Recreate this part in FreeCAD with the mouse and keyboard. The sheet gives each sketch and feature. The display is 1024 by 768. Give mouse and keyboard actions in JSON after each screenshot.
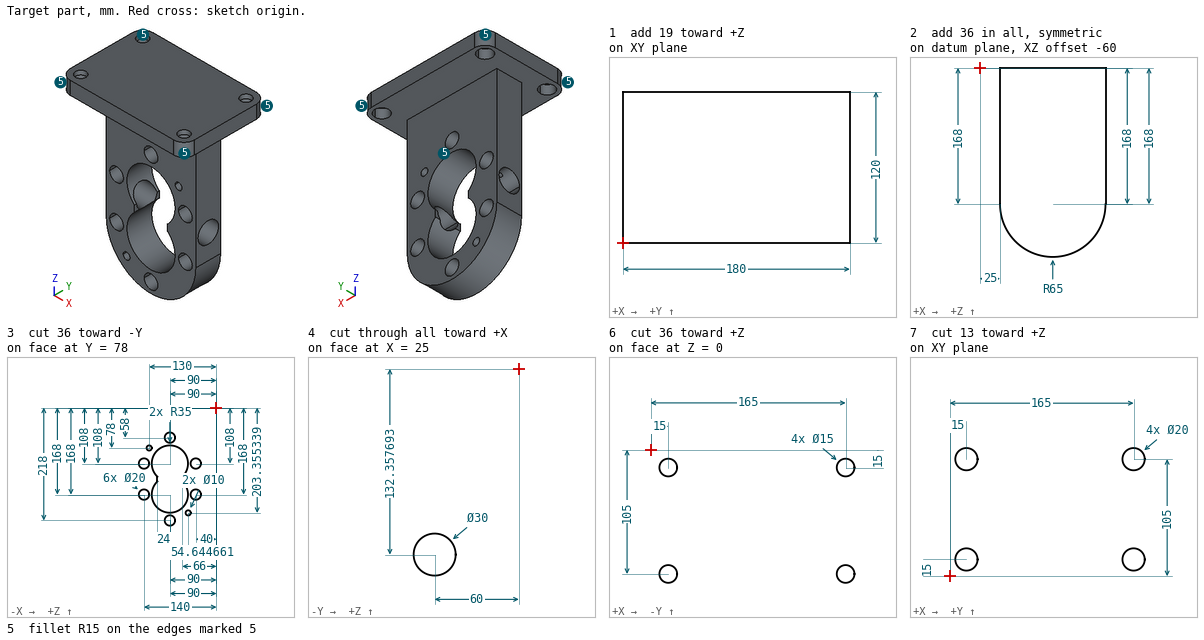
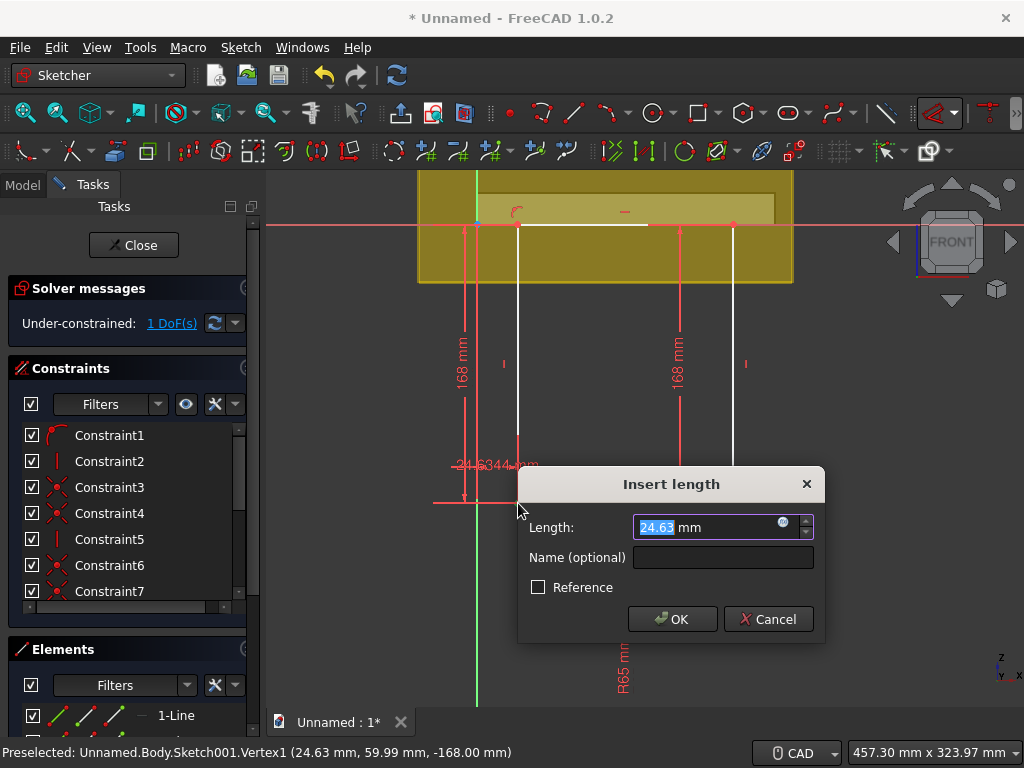
{"action": "type", "text": "25"}
{"action": "key", "text": "Return"}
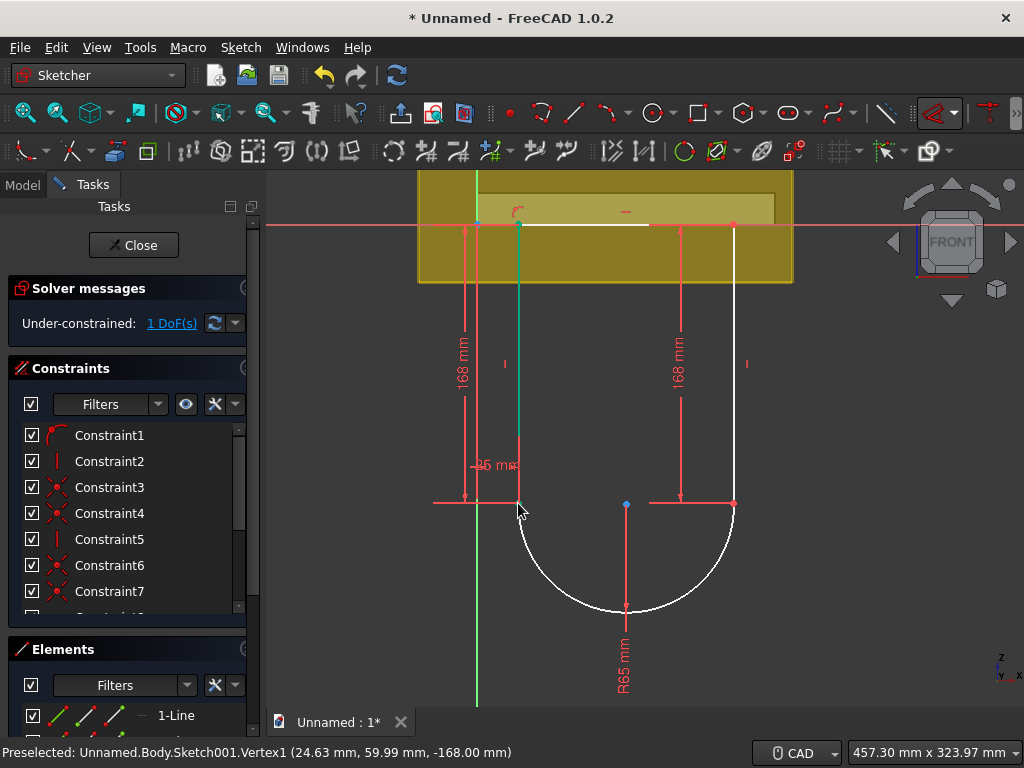
{"action": "left_click", "coordinate": [626, 505]}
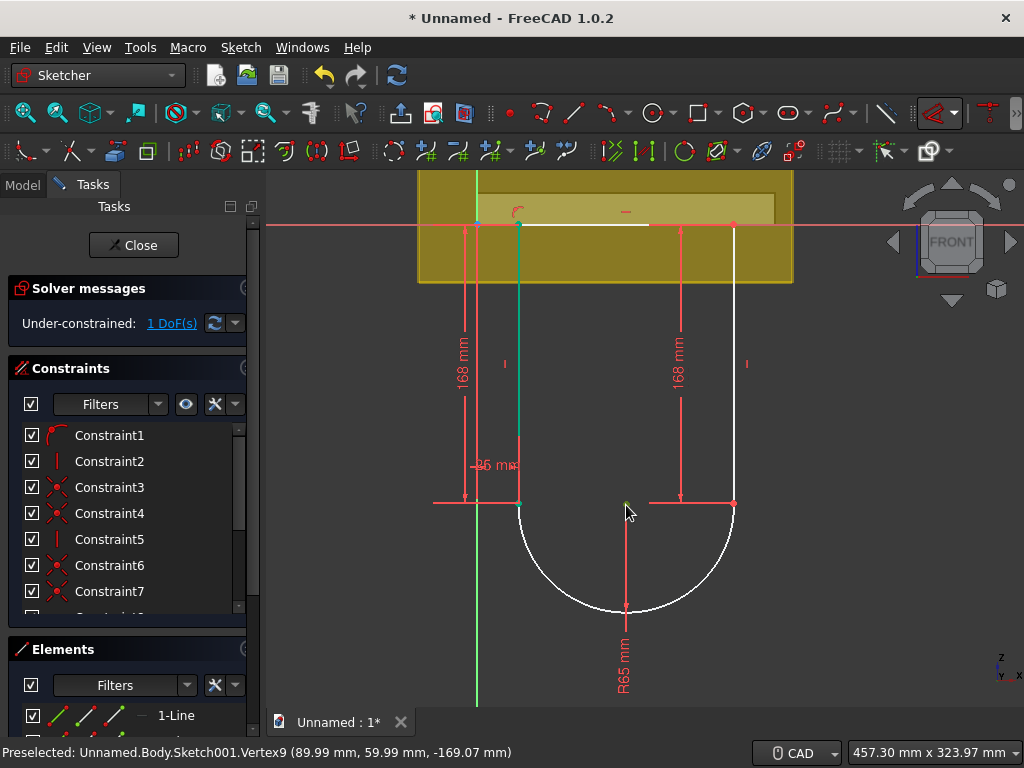
{"action": "left_click", "coordinate": [956, 114]}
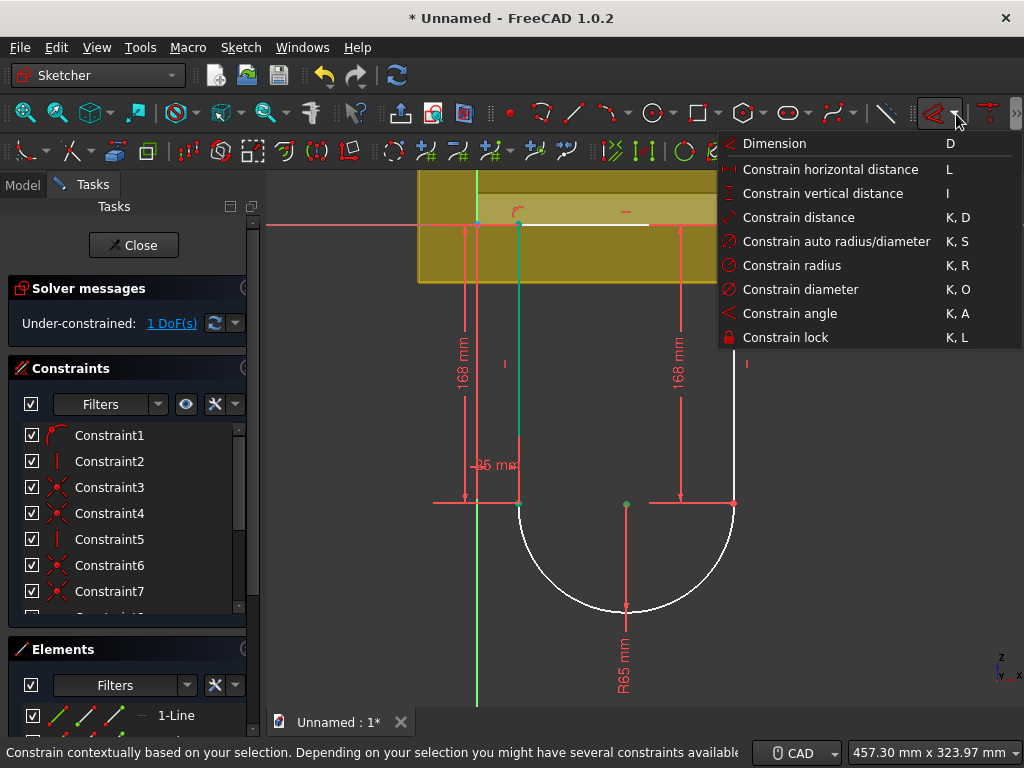
{"action": "left_click", "coordinate": [870, 193]}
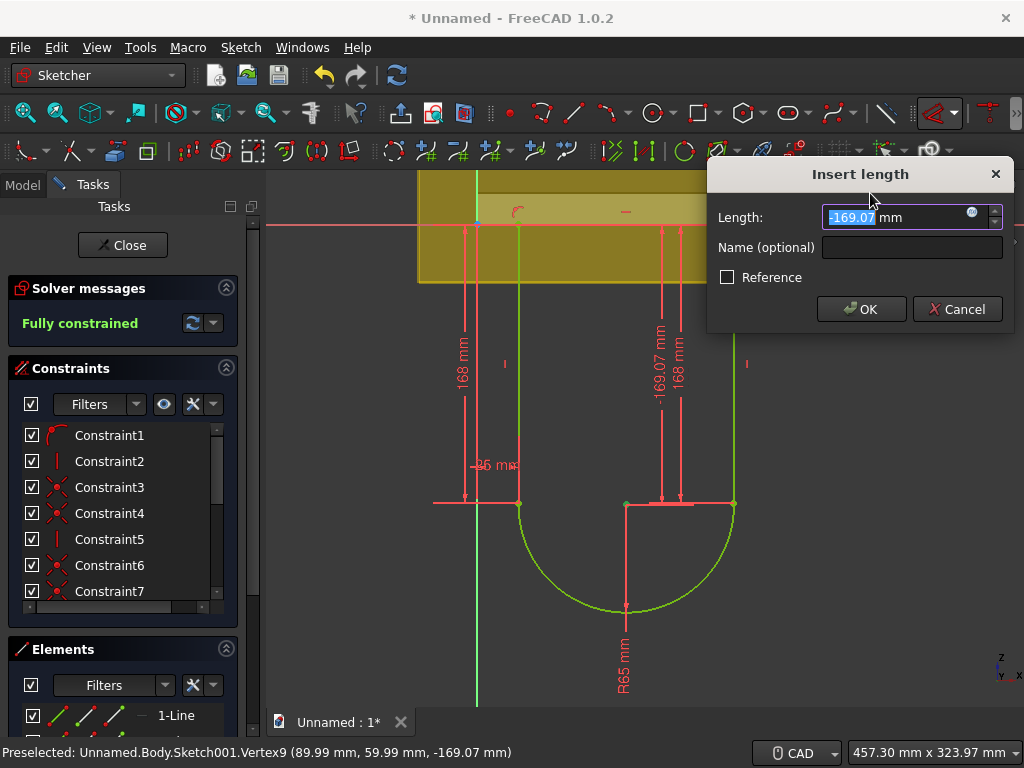
{"action": "type", "text": "-168"}
{"action": "key", "text": "Return"}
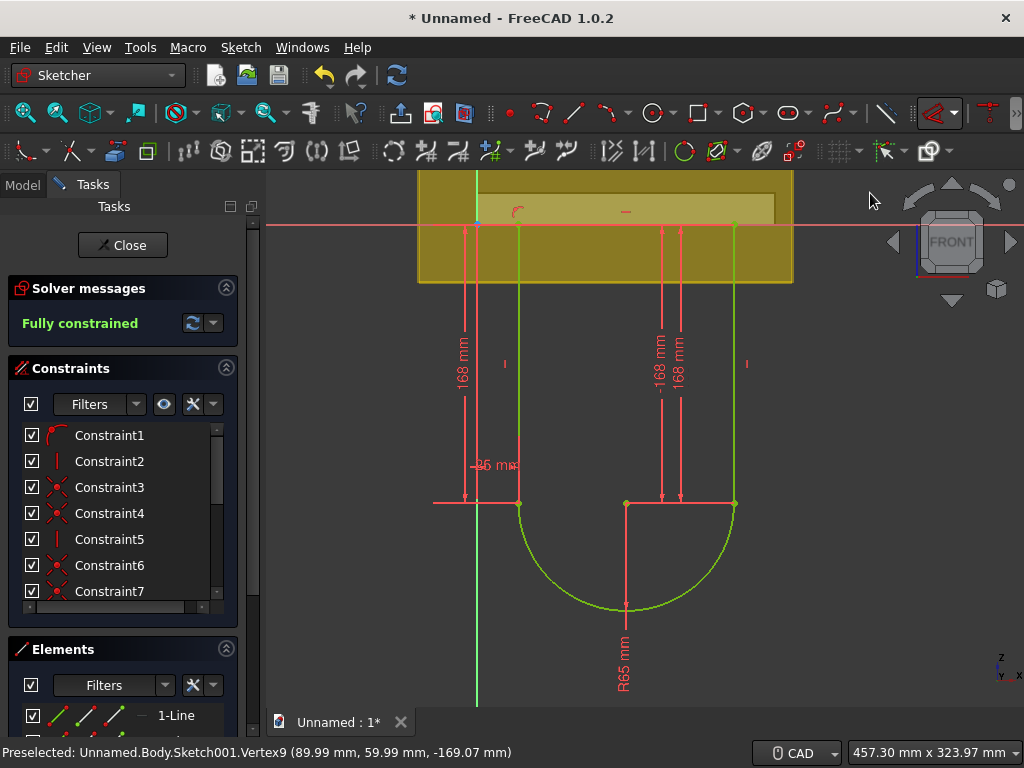
{"action": "left_click", "coordinate": [123, 245]}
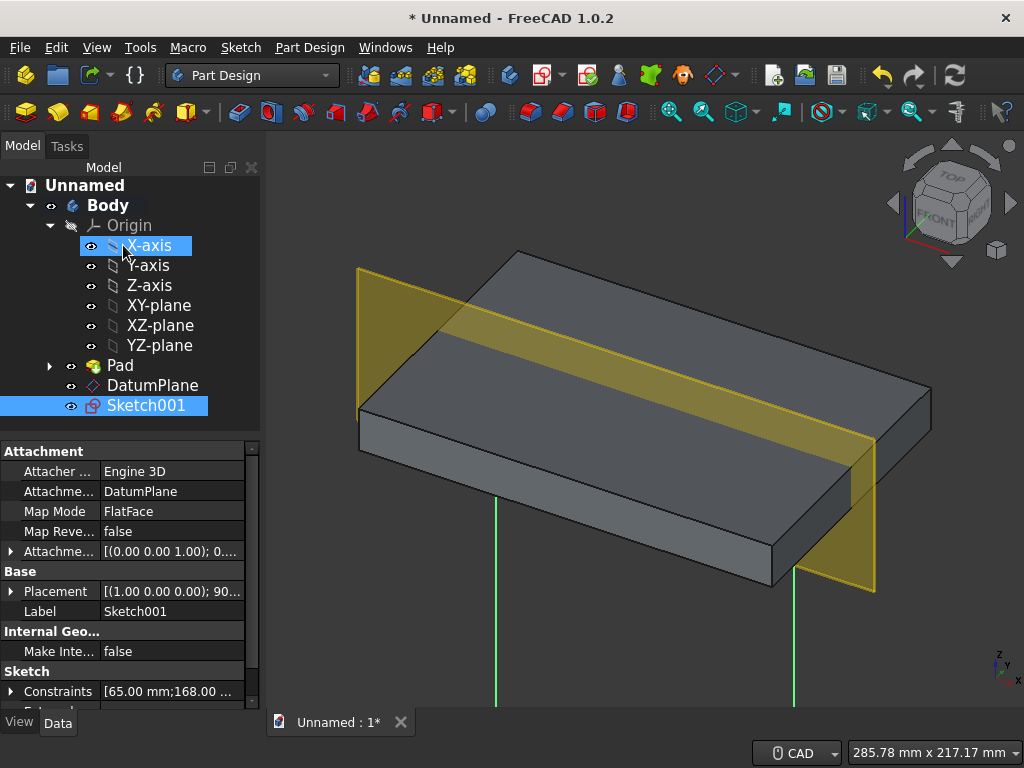
{"action": "left_click", "coordinate": [26, 112]}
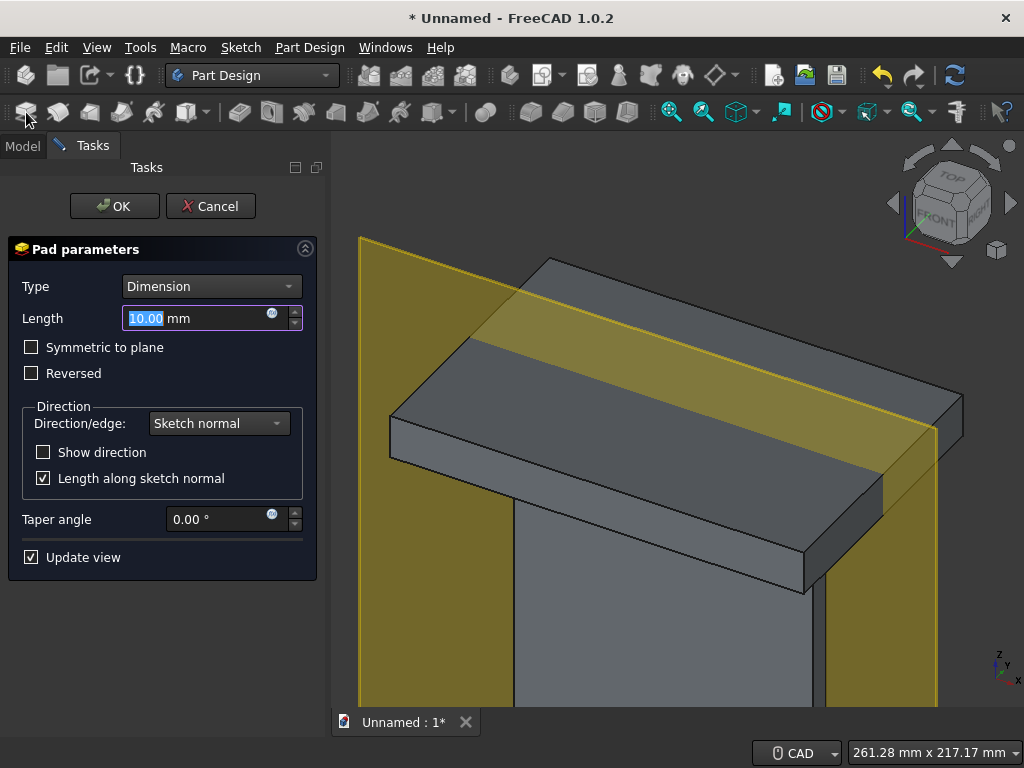
{"action": "type", "text": "36"}
{"action": "key", "text": "Tab"}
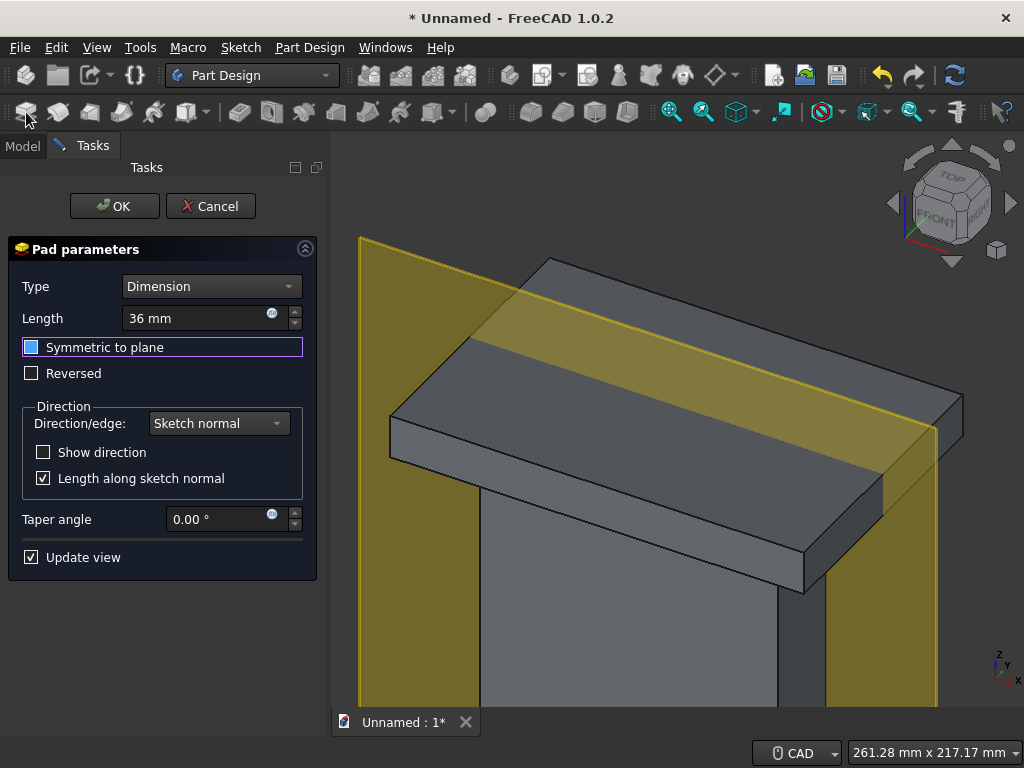
{"action": "left_click", "coordinate": [30, 347]}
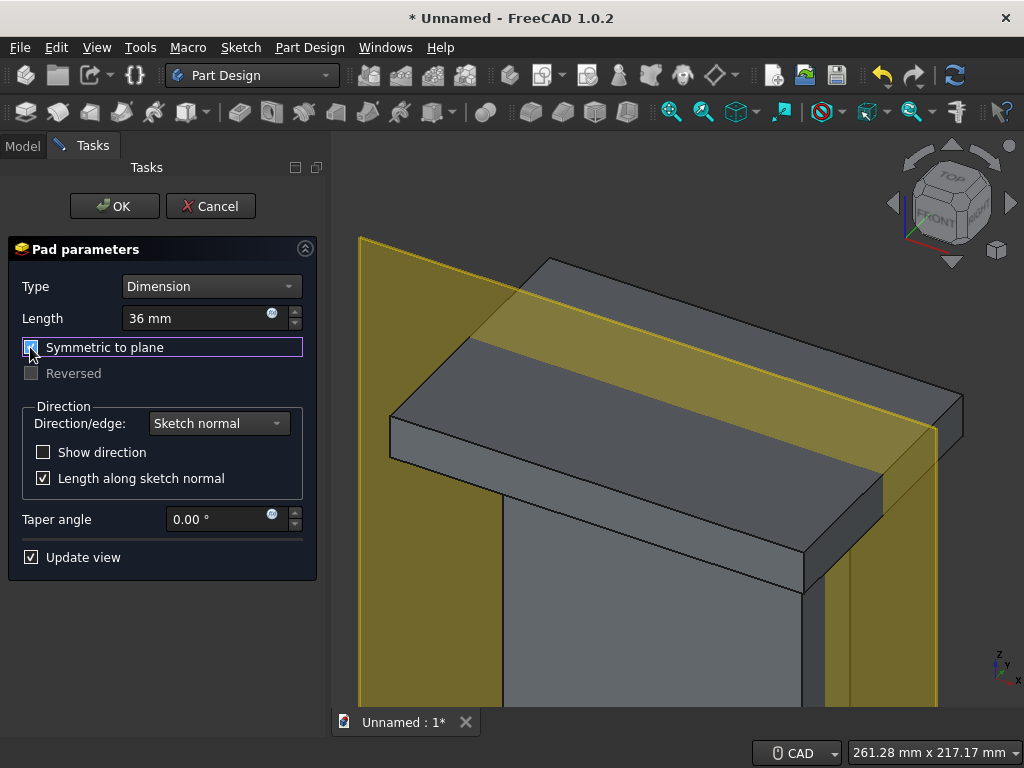
{"action": "left_click", "coordinate": [115, 206]}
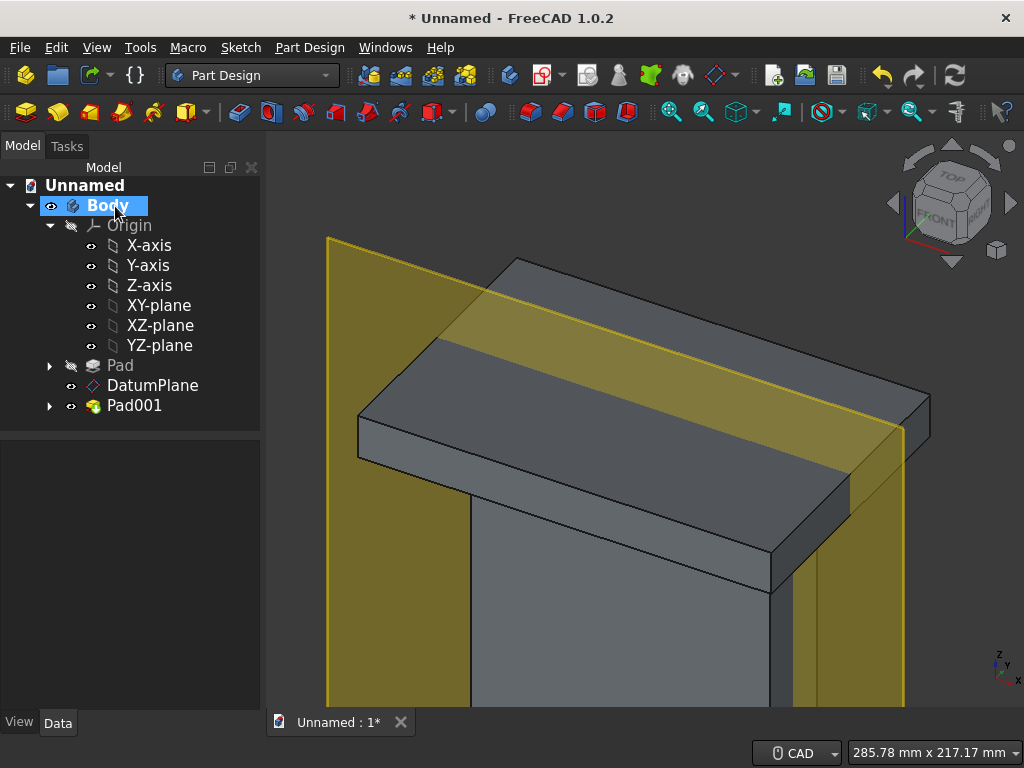
{"action": "left_click", "coordinate": [116, 386]}
{"action": "key", "text": "space"}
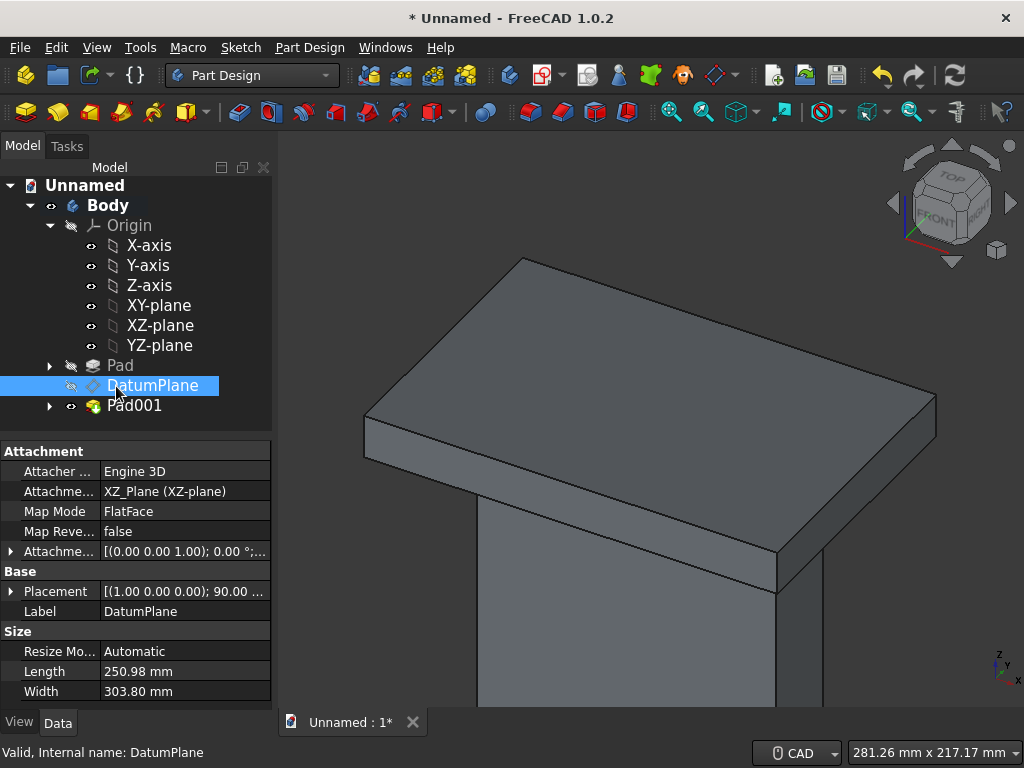
{"action": "left_click", "coordinate": [672, 112]}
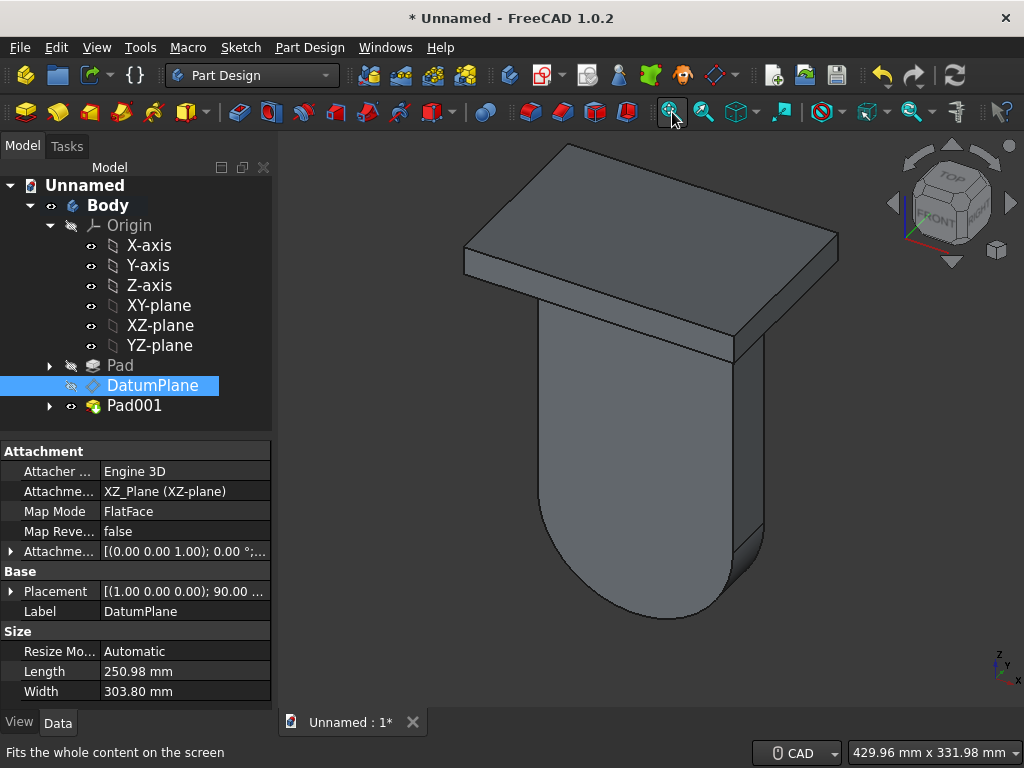
{"action": "key", "text": "4"}